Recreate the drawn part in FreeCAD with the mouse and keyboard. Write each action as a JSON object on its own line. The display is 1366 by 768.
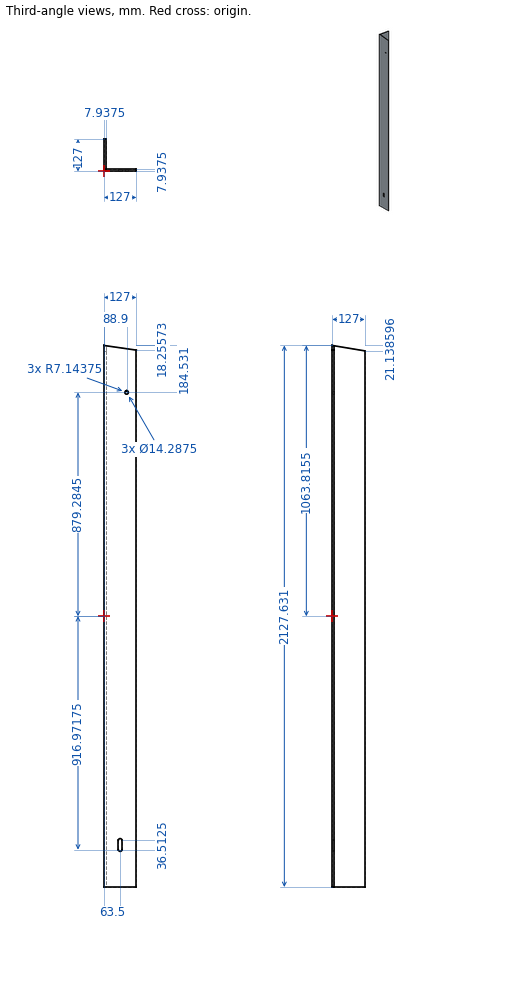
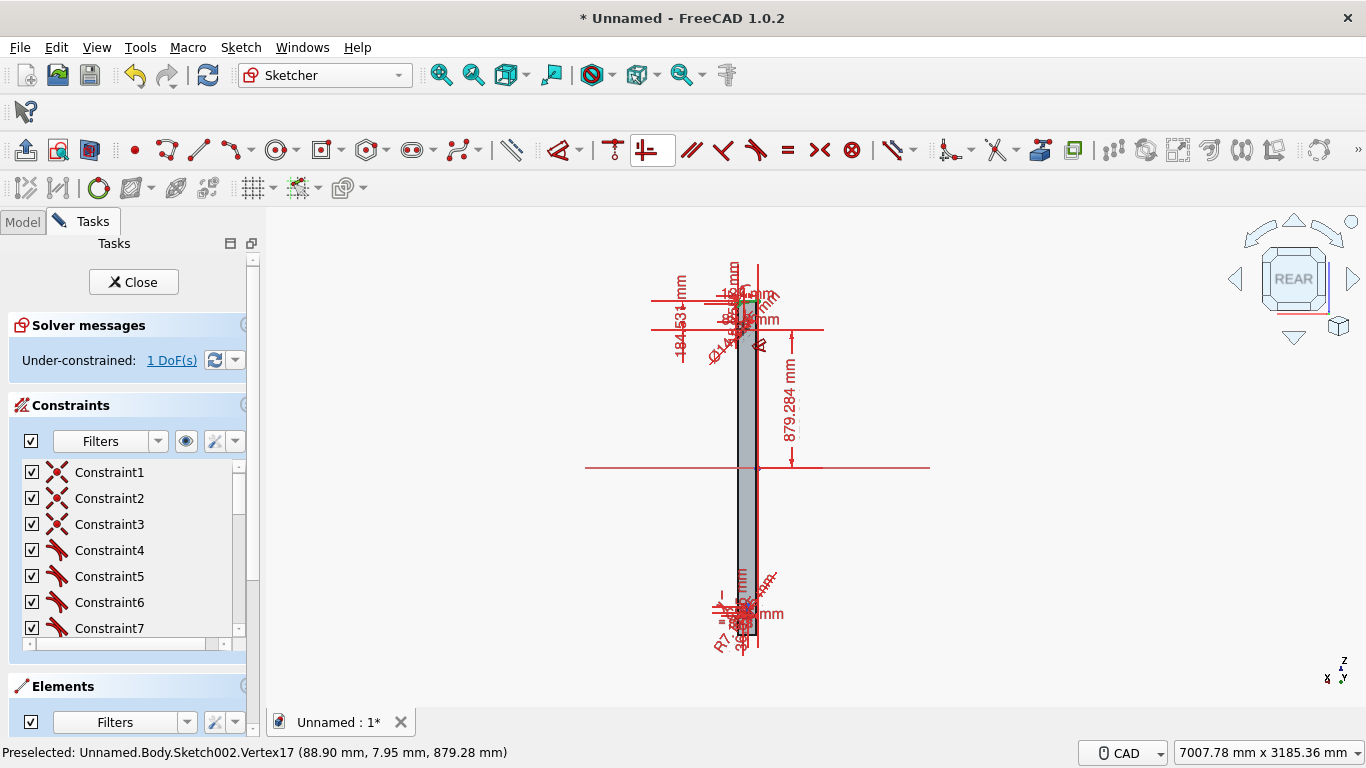
{"action": "scroll", "coordinate": [747, 613], "scroll_direction": "up", "scroll_amount": 12}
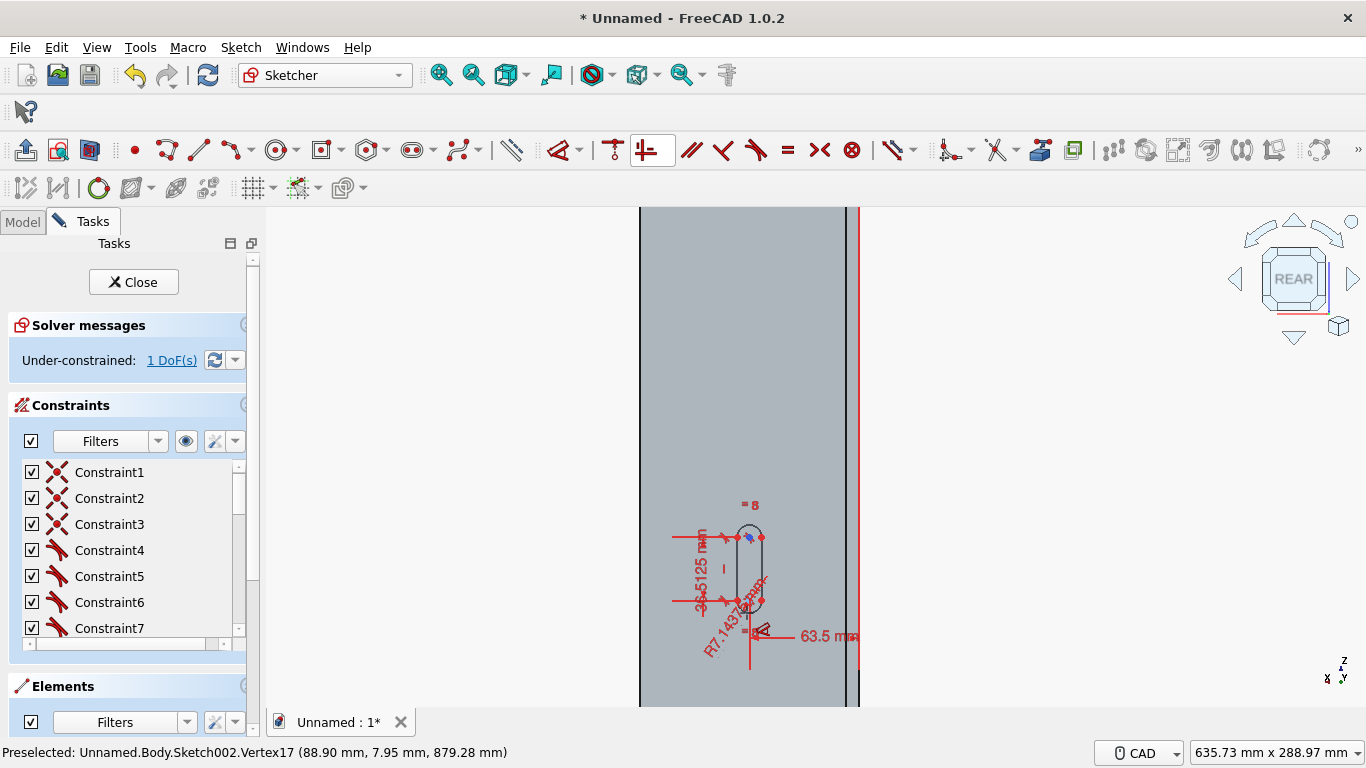
{"action": "left_click", "coordinate": [737, 601]}
{"action": "left_click", "coordinate": [893, 418]}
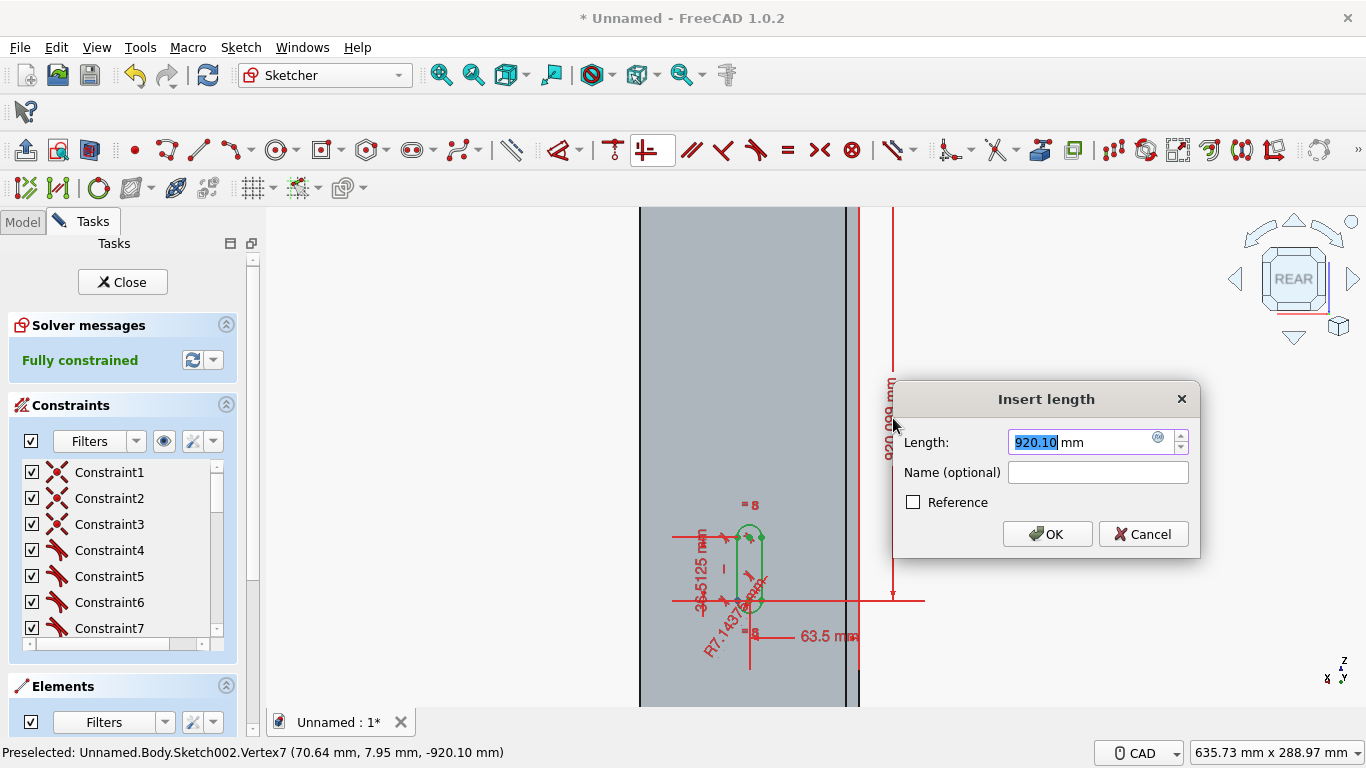
{"action": "type", "text": "916.97175"}
{"action": "key", "text": "Return"}
{"action": "key", "text": "Escape"}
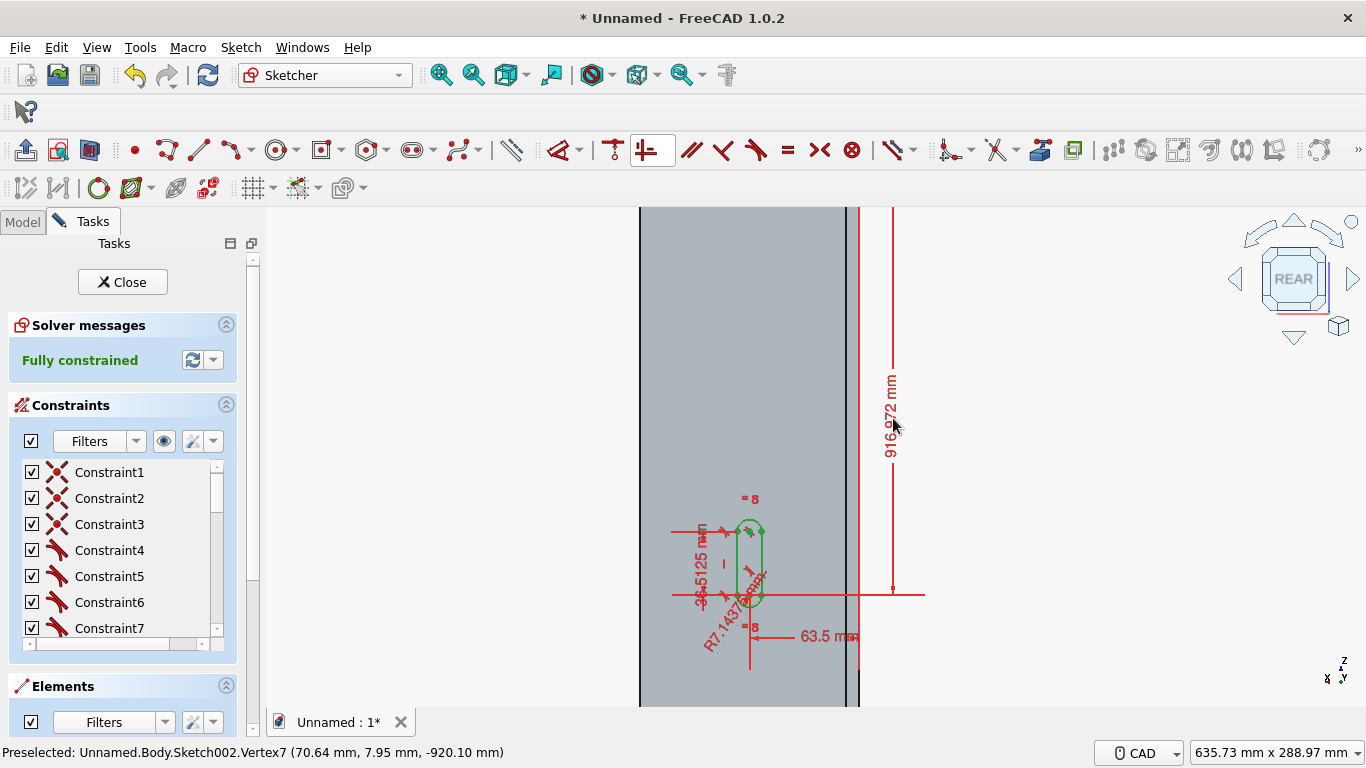
{"action": "left_click", "coordinate": [123, 282]}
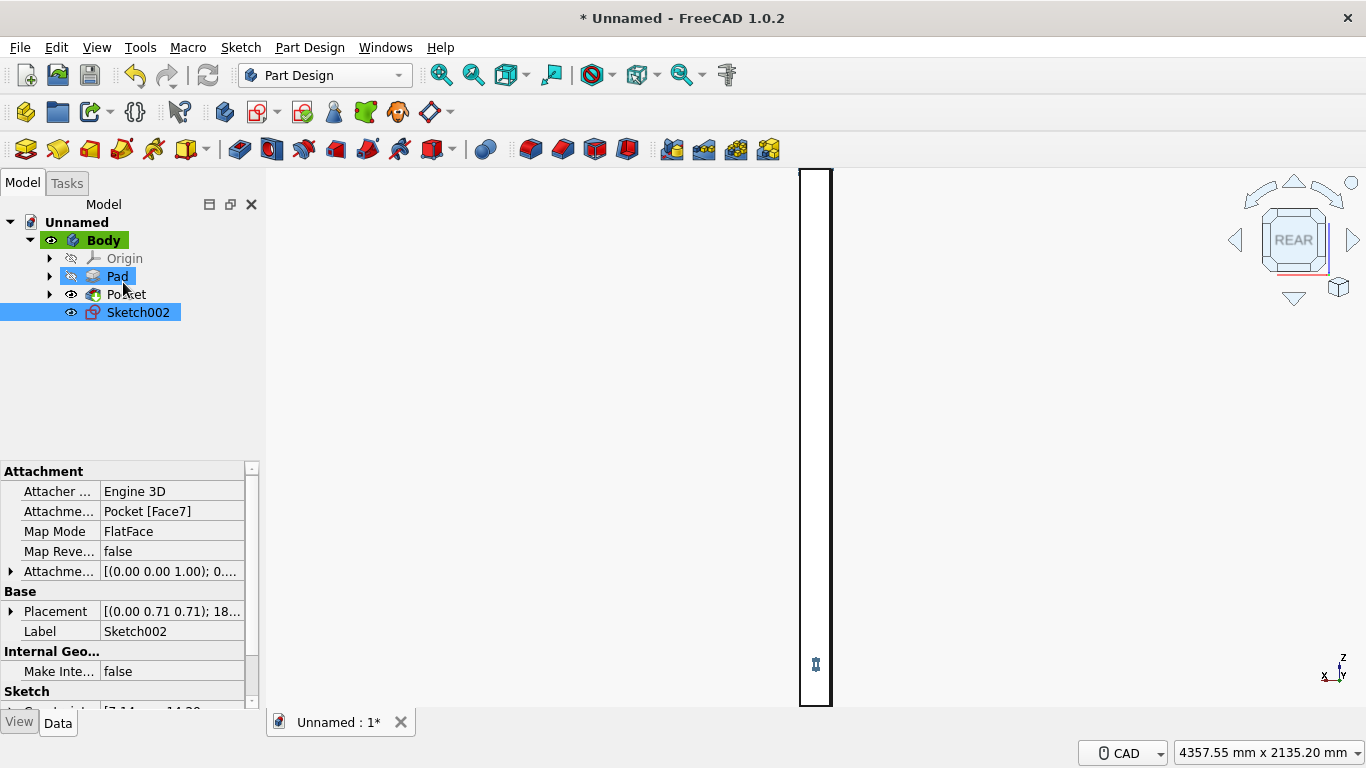
{"action": "left_click", "coordinate": [240, 150]}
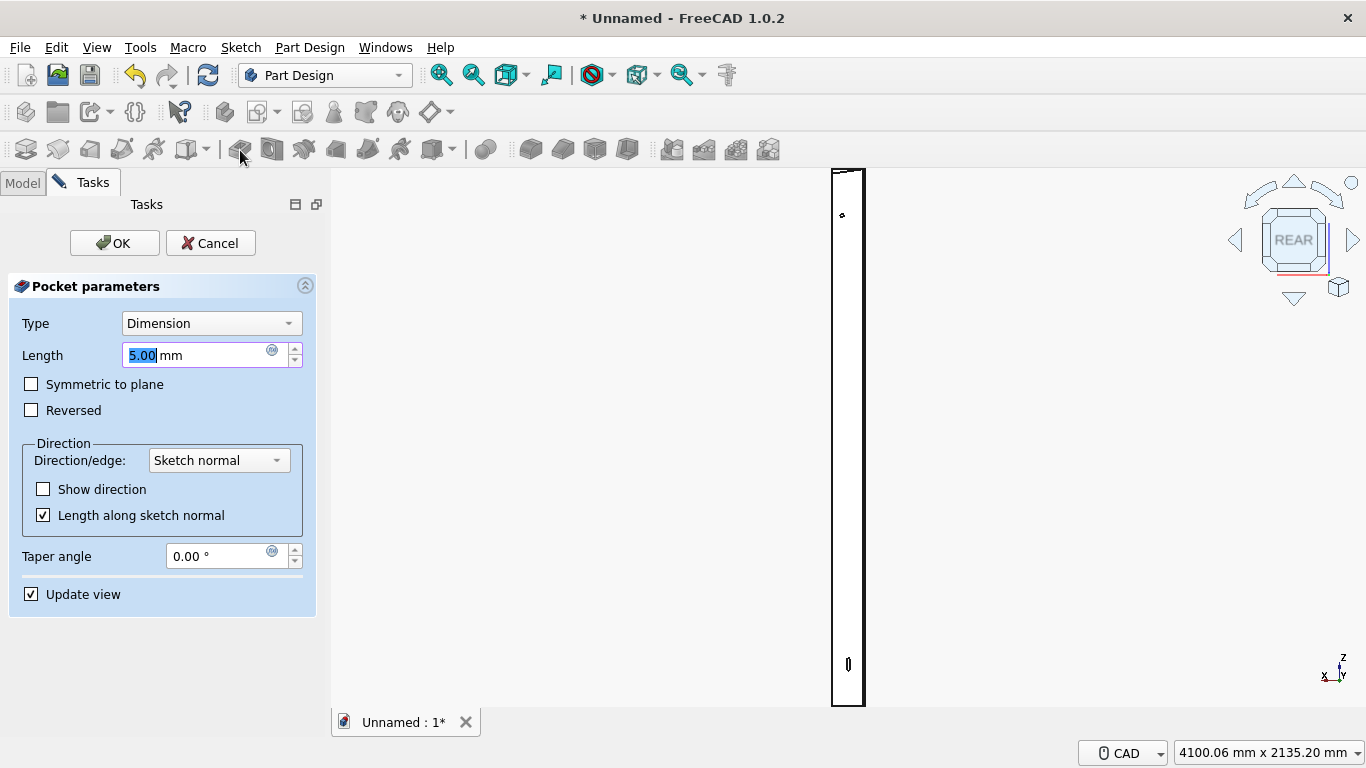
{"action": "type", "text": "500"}
{"action": "key", "text": "Tab"}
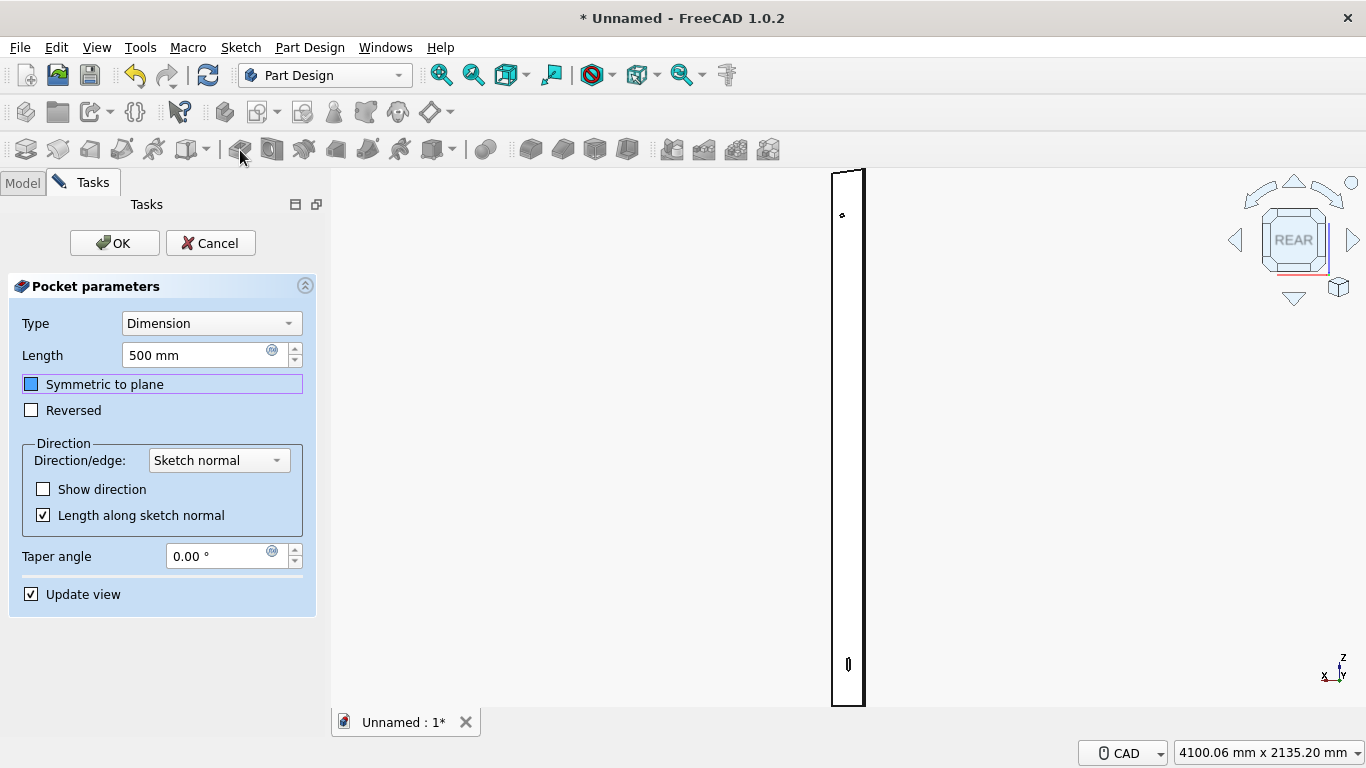
{"action": "left_click", "coordinate": [30, 384]}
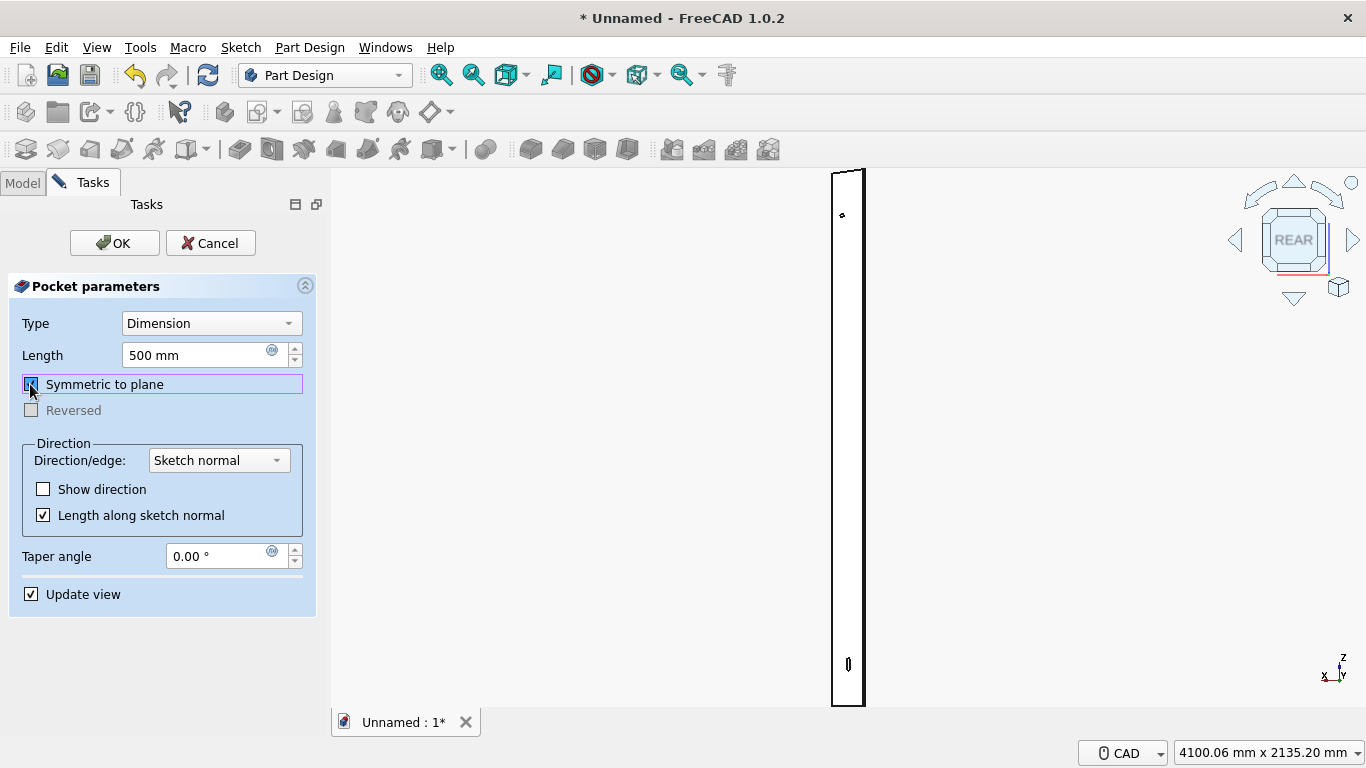
{"action": "left_click", "coordinate": [115, 243]}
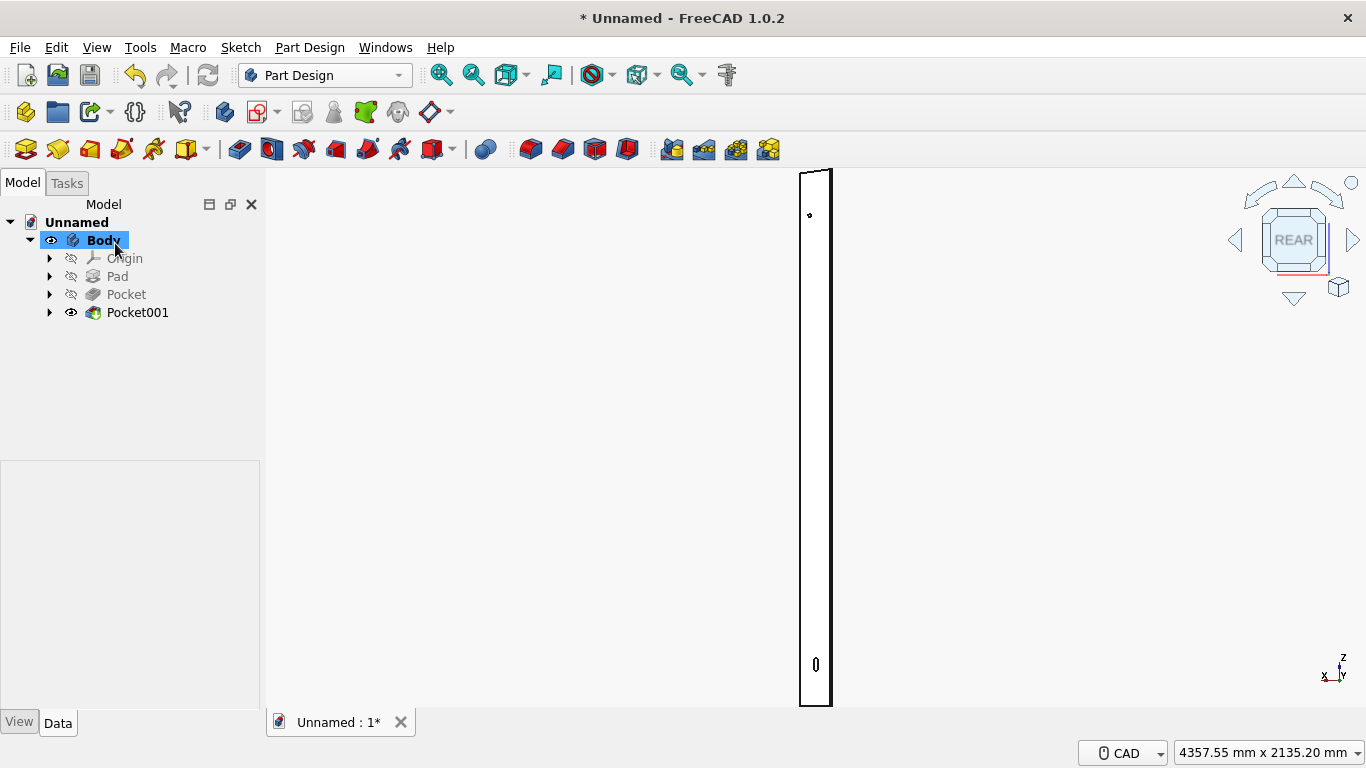
{"action": "key", "text": "0"}